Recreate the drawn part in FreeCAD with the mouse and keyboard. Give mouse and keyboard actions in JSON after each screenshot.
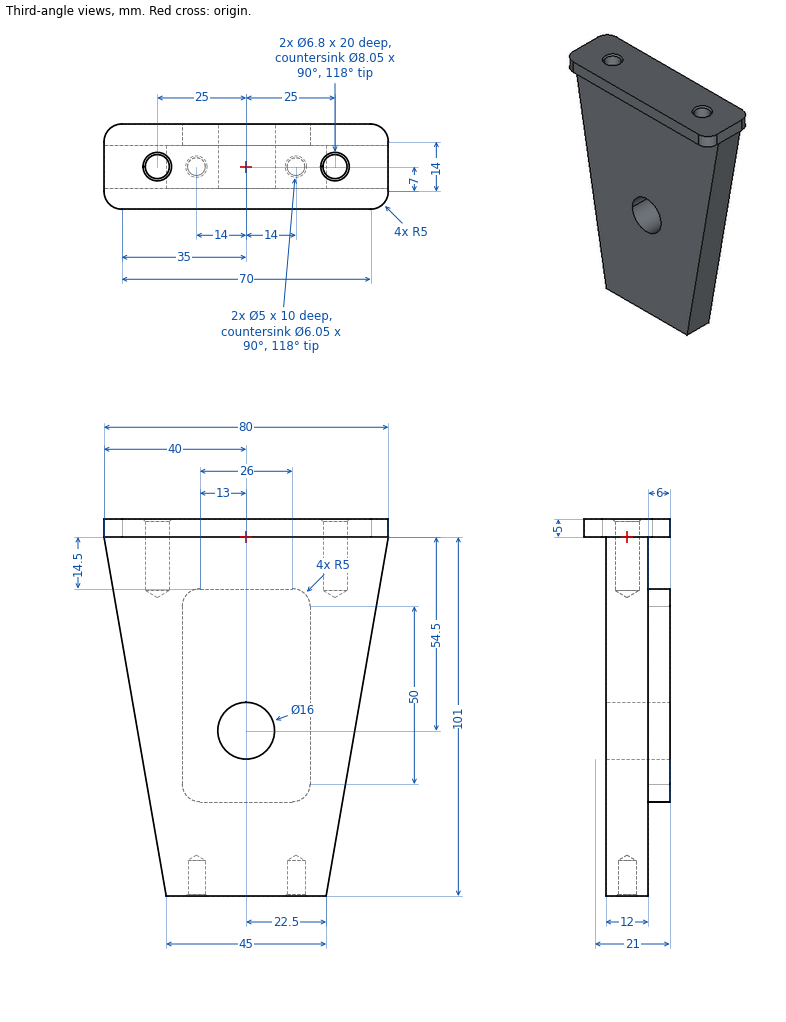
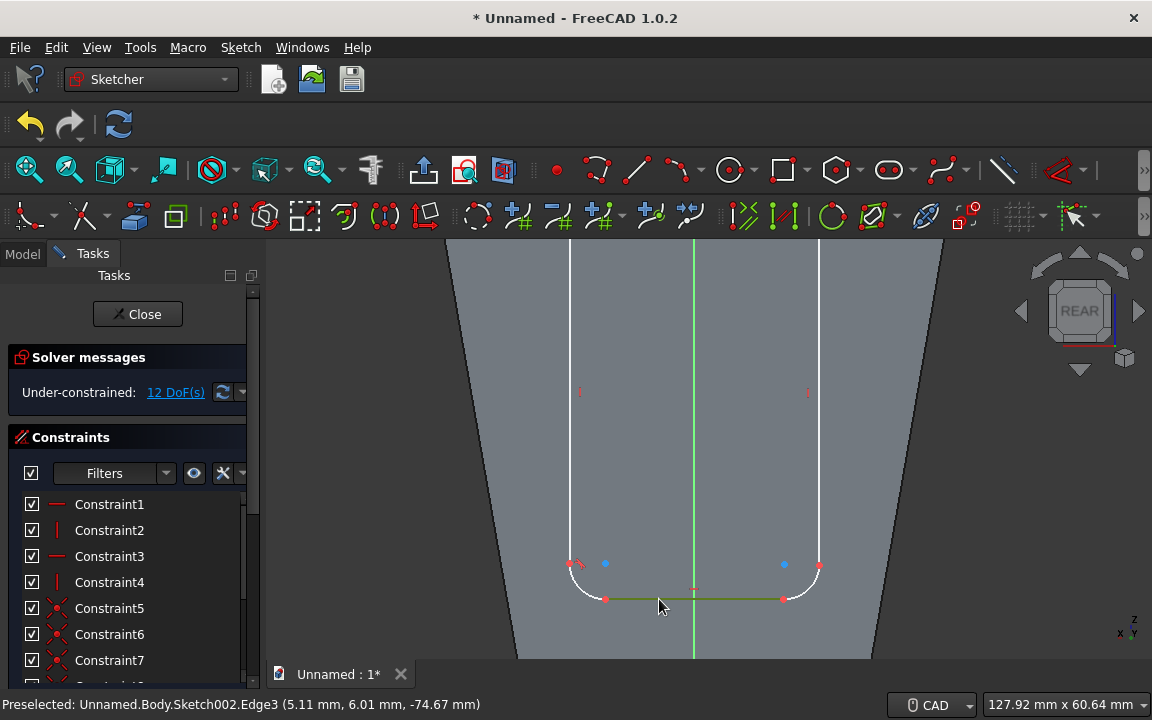
{"action": "left_click", "coordinate": [574, 580]}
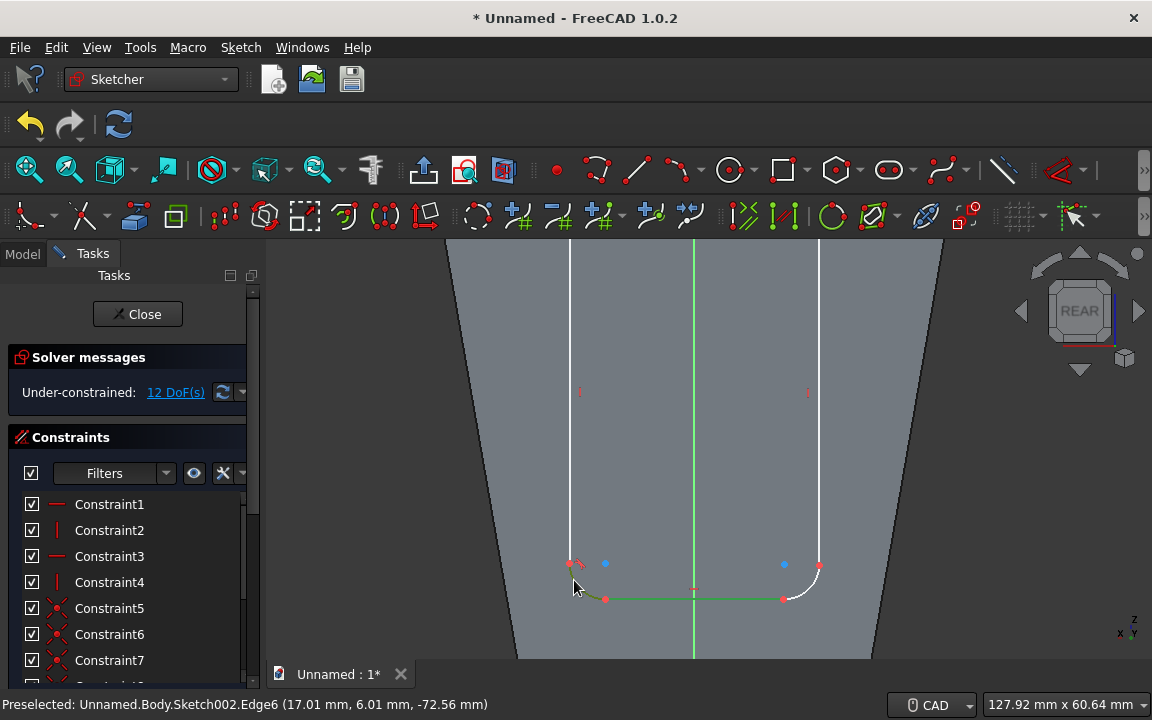
{"action": "key", "text": "t"}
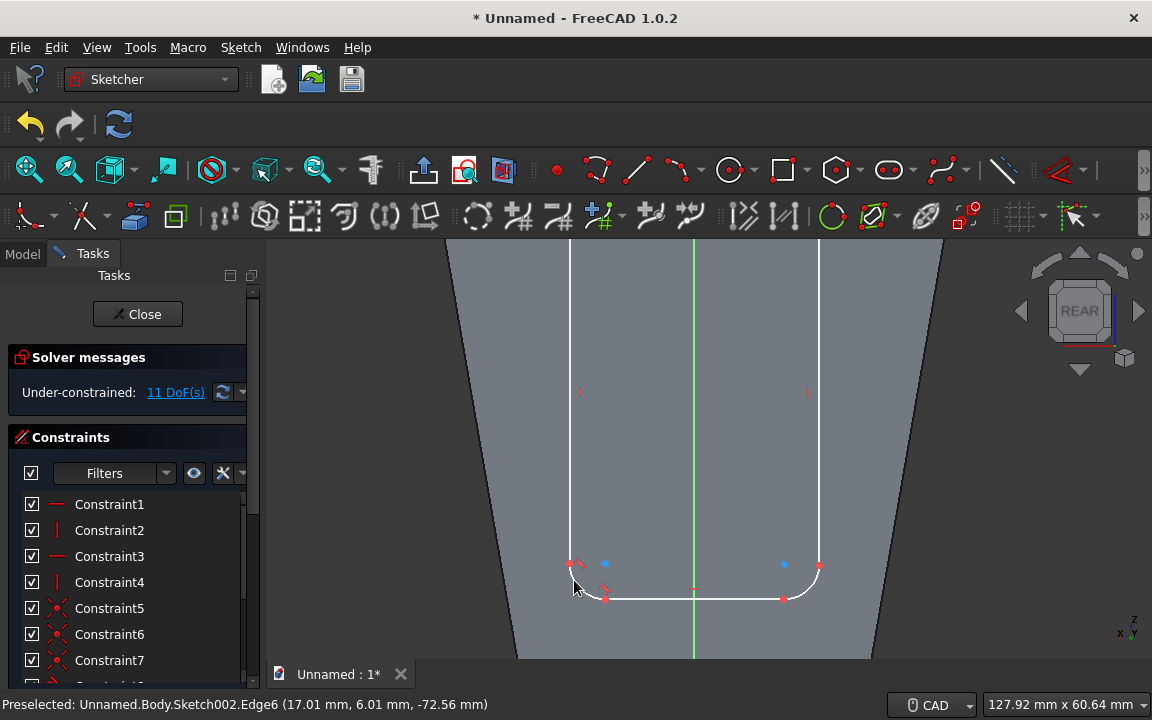
{"action": "left_click", "coordinate": [659, 599]}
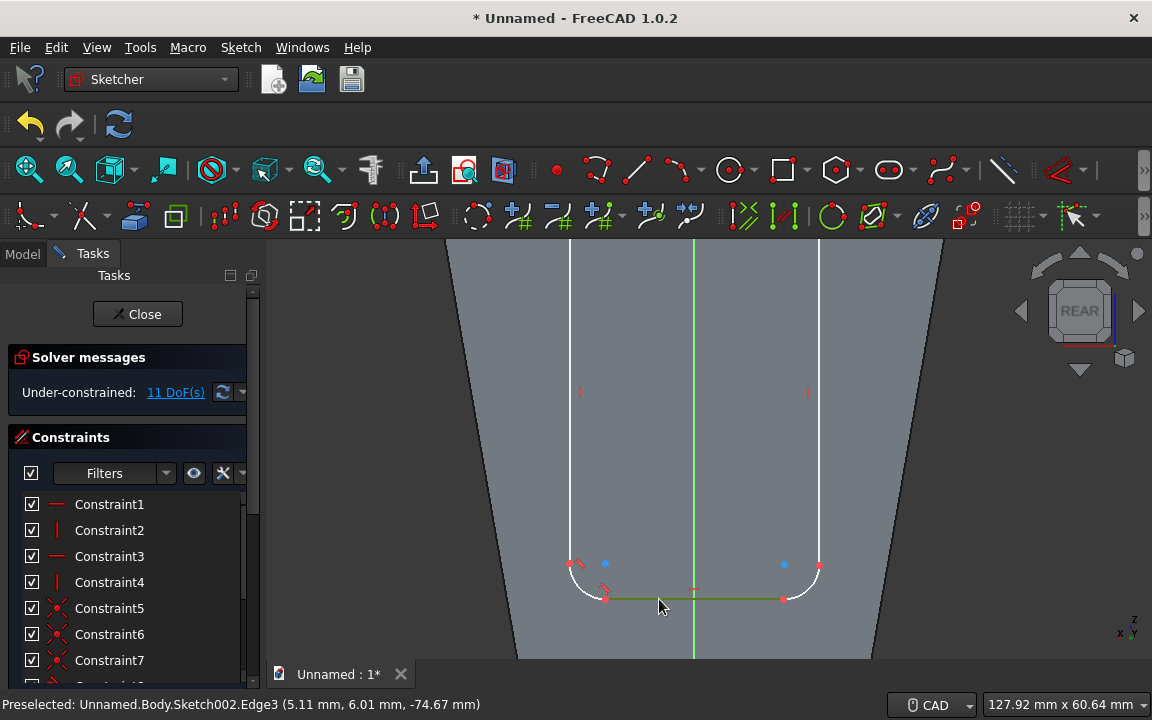
{"action": "left_click", "coordinate": [799, 596]}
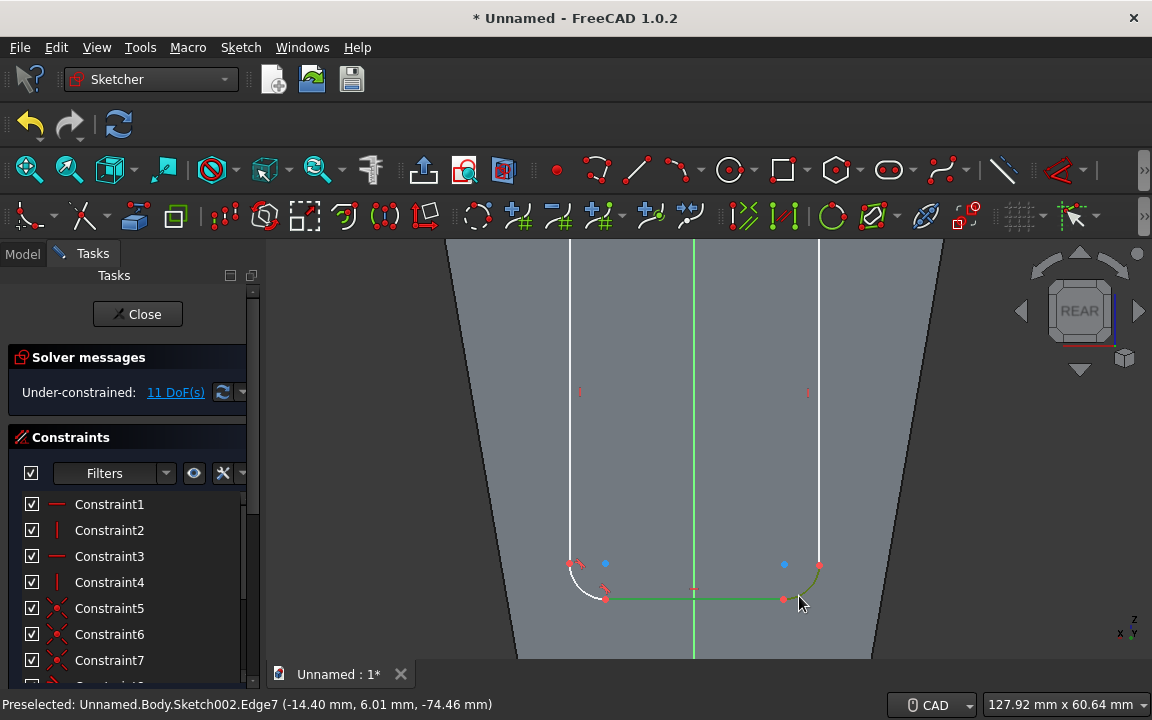
{"action": "key", "text": "t"}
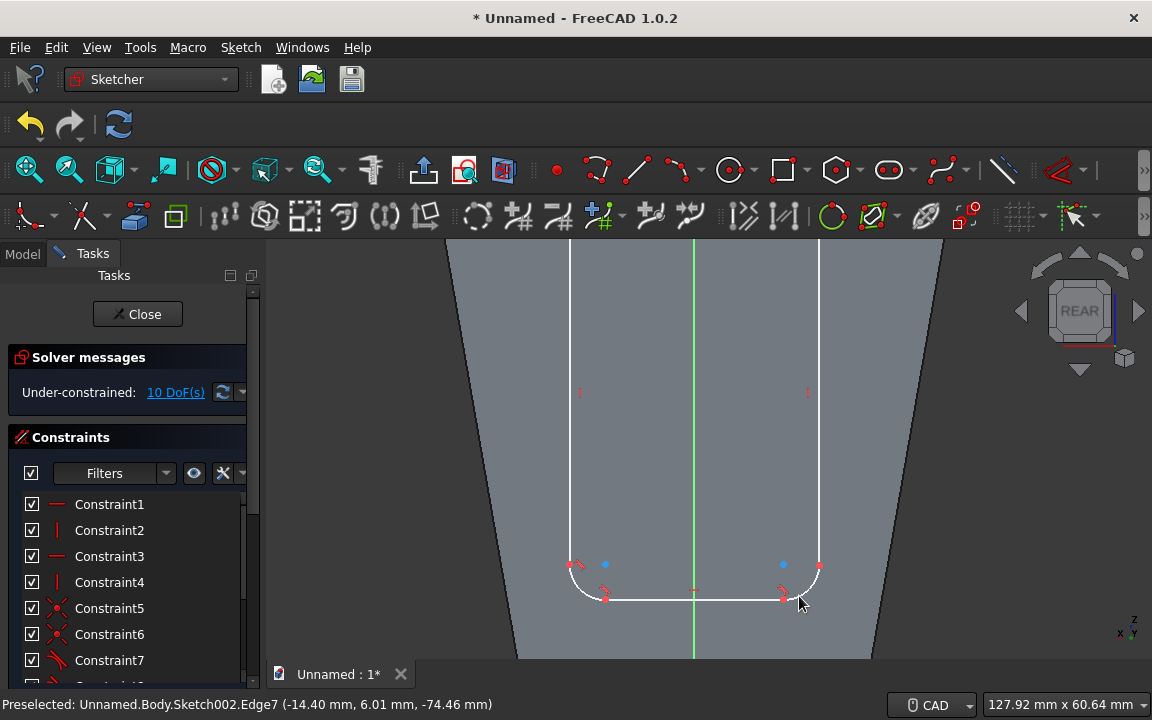
{"action": "left_click", "coordinate": [819, 462]}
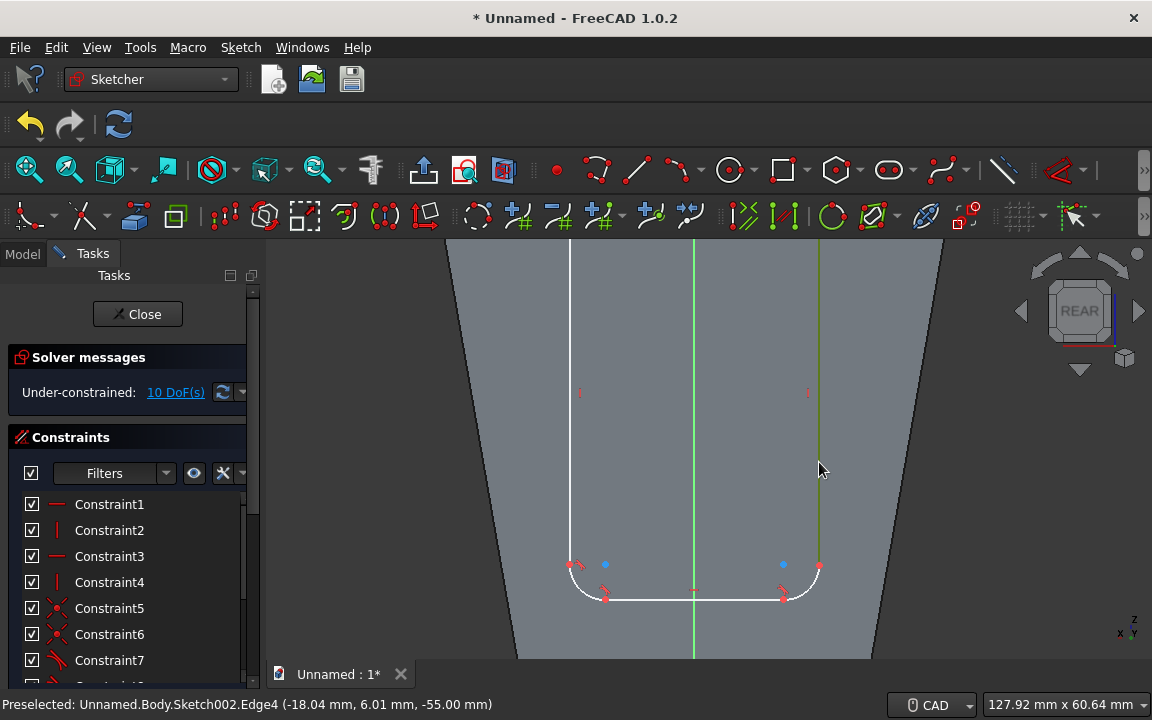
{"action": "left_click", "coordinate": [799, 596]}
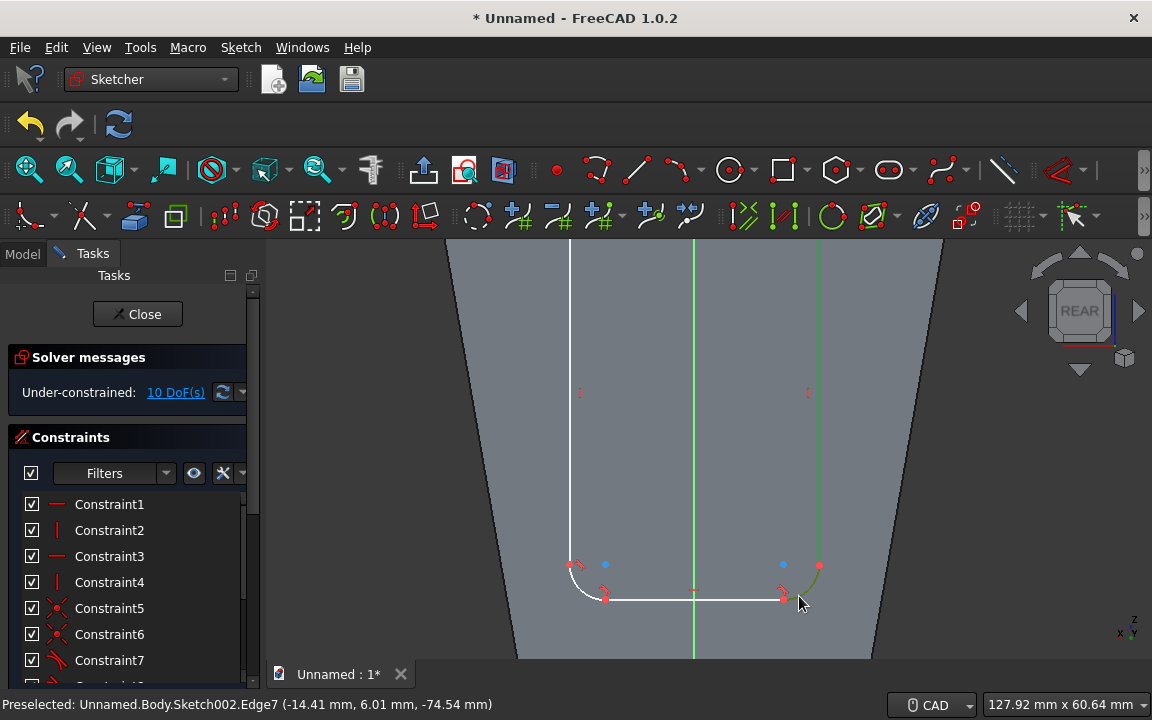
{"action": "key", "text": "t"}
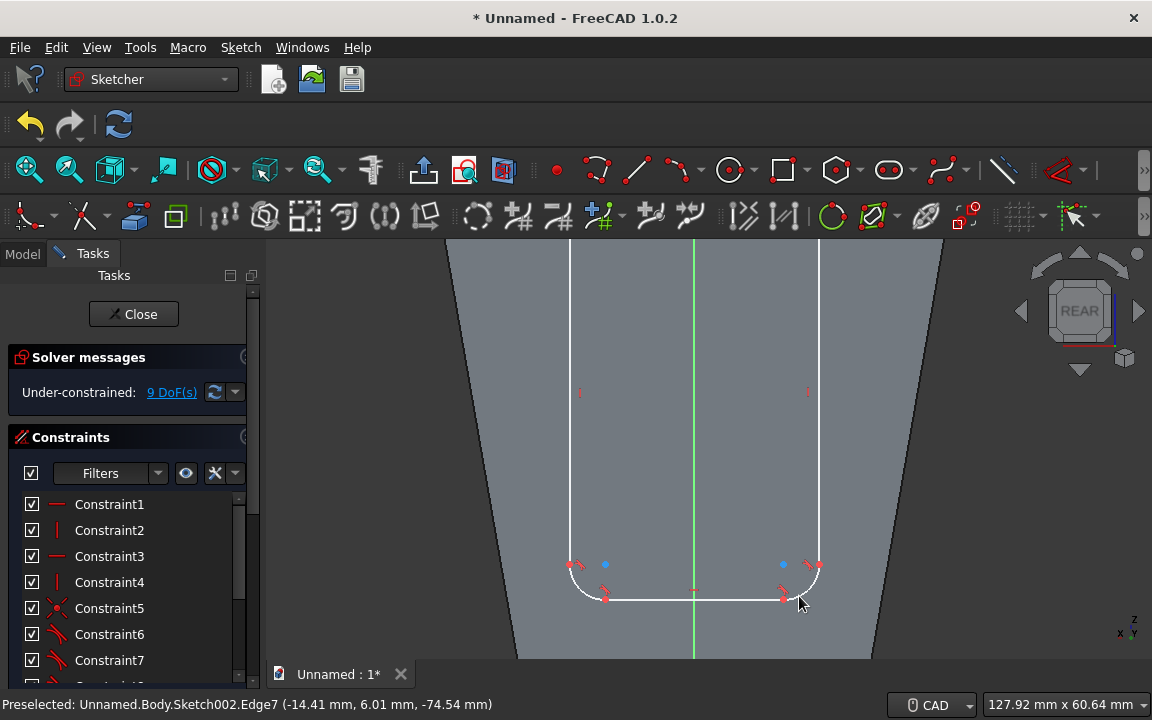
{"action": "left_click", "coordinate": [819, 460]}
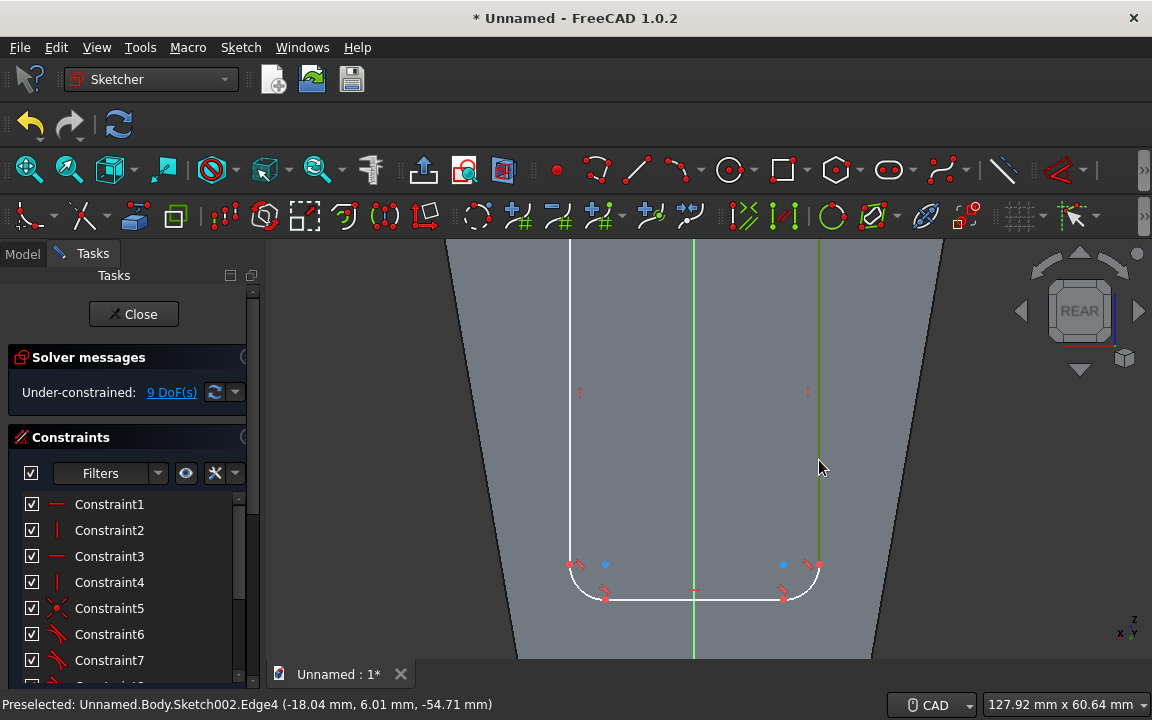
{"action": "scroll", "coordinate": [575, 582], "scroll_direction": "down", "scroll_amount": 3}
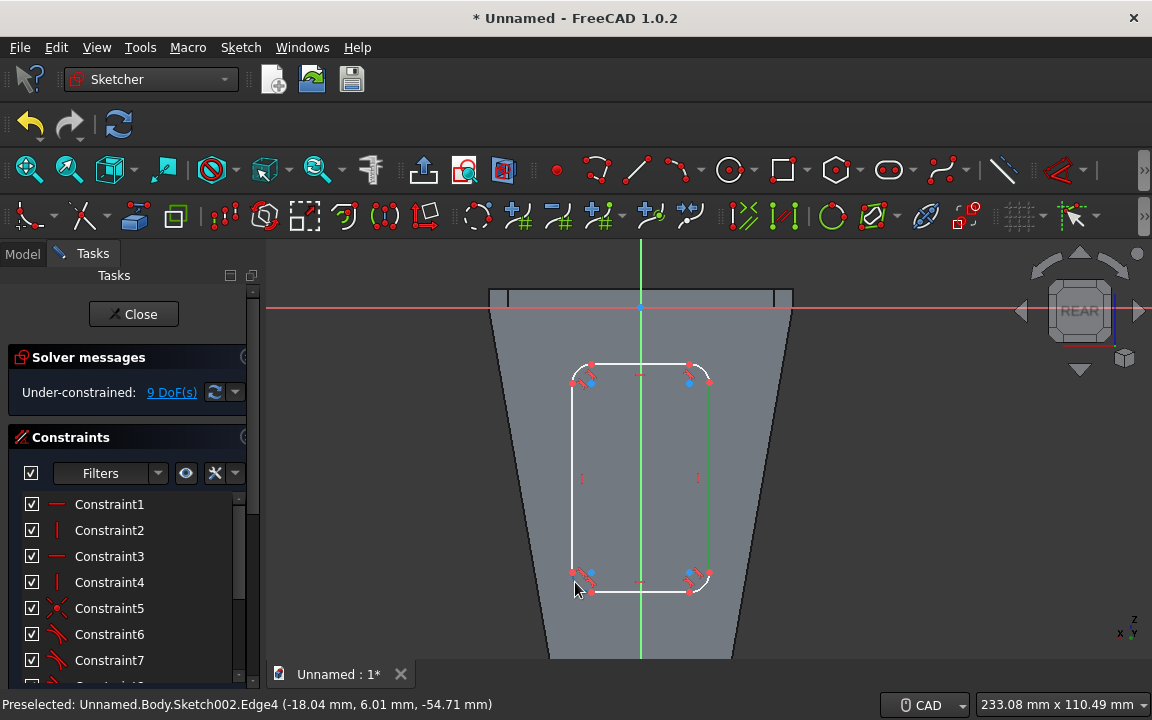
{"action": "scroll", "coordinate": [707, 374], "scroll_direction": "up", "scroll_amount": 3}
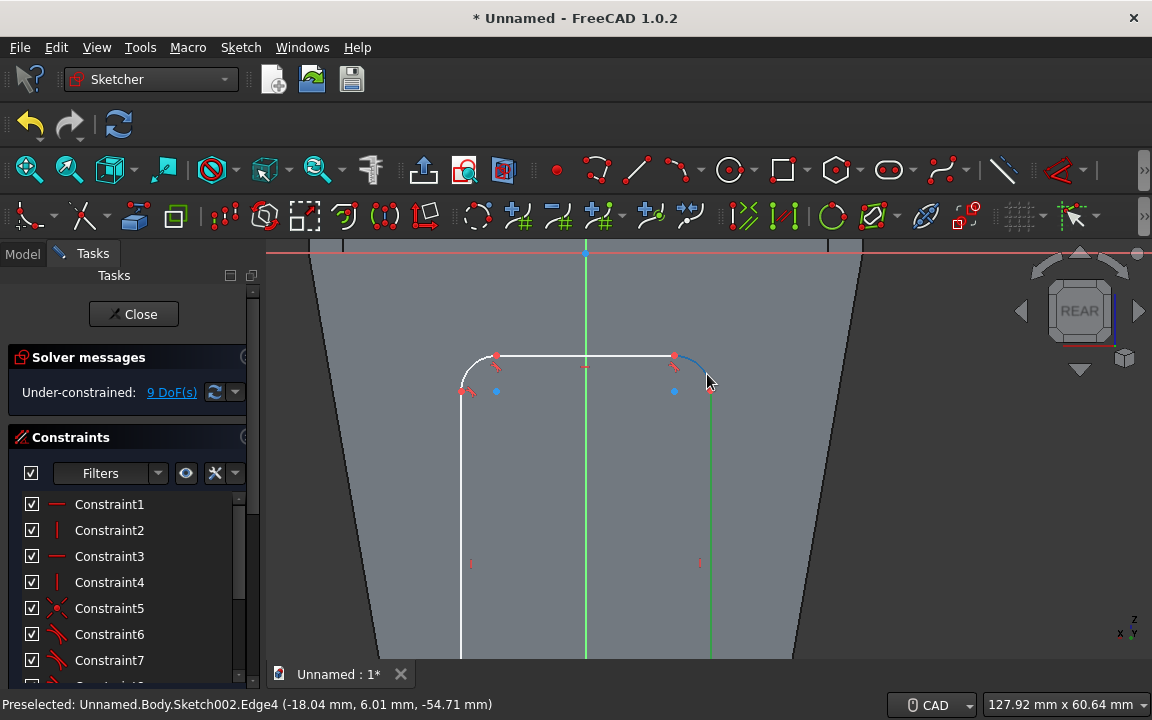
{"action": "left_click", "coordinate": [706, 374]}